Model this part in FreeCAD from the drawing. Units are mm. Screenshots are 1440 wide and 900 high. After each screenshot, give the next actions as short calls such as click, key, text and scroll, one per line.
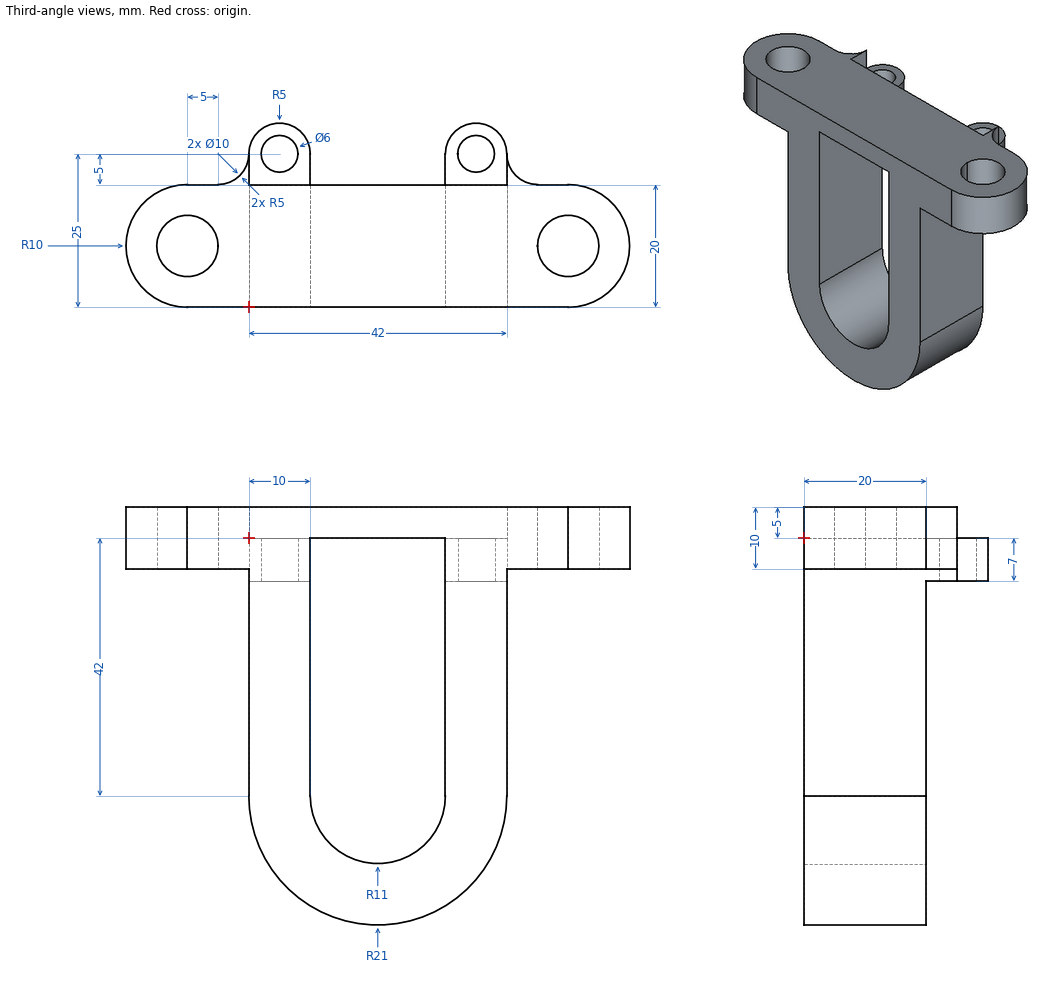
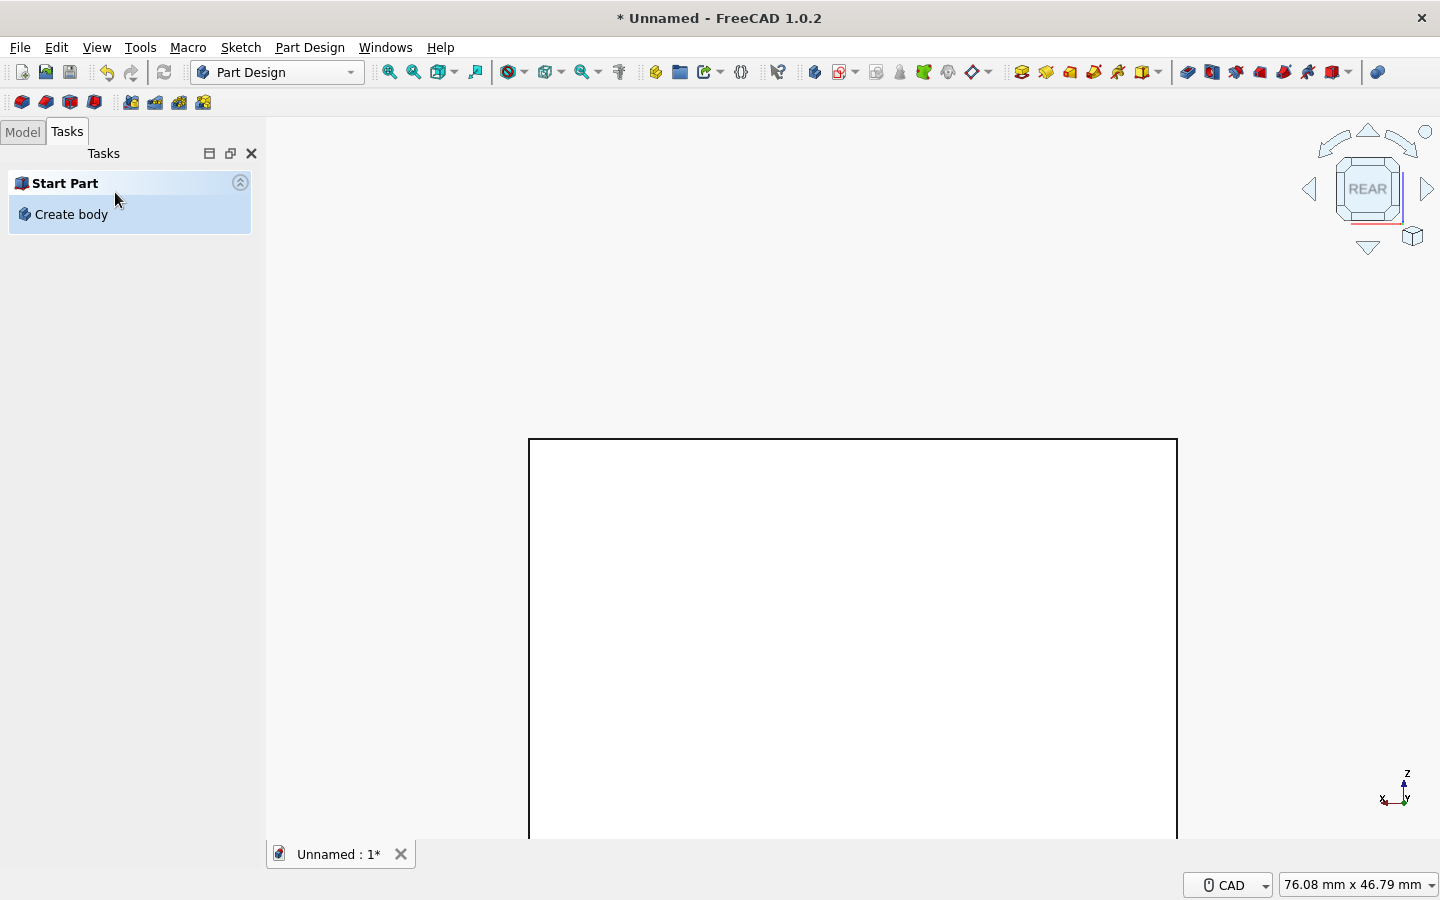
click(390, 72)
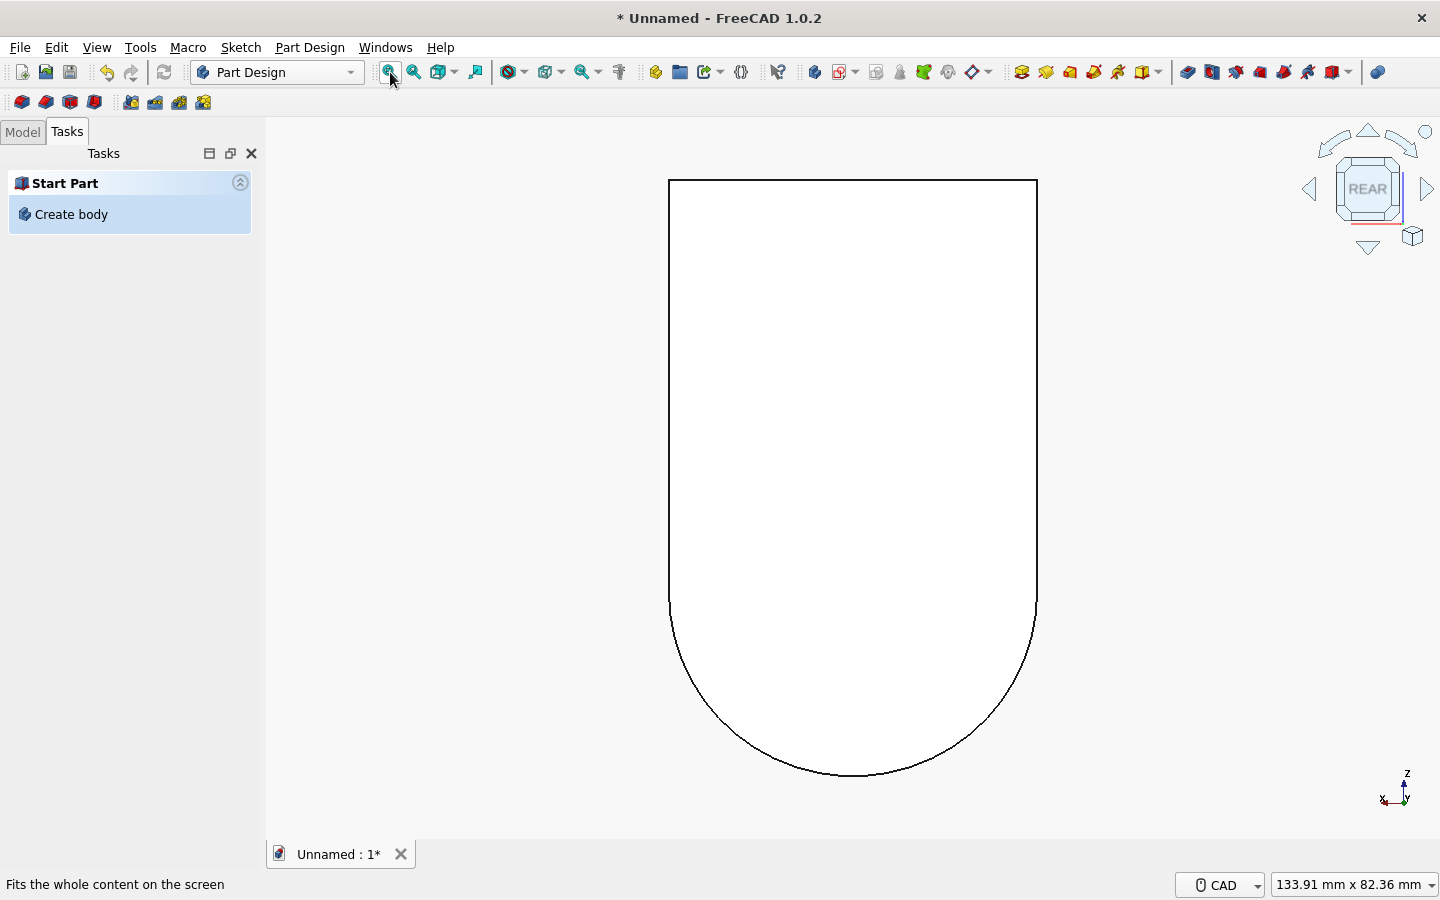
click(853, 392)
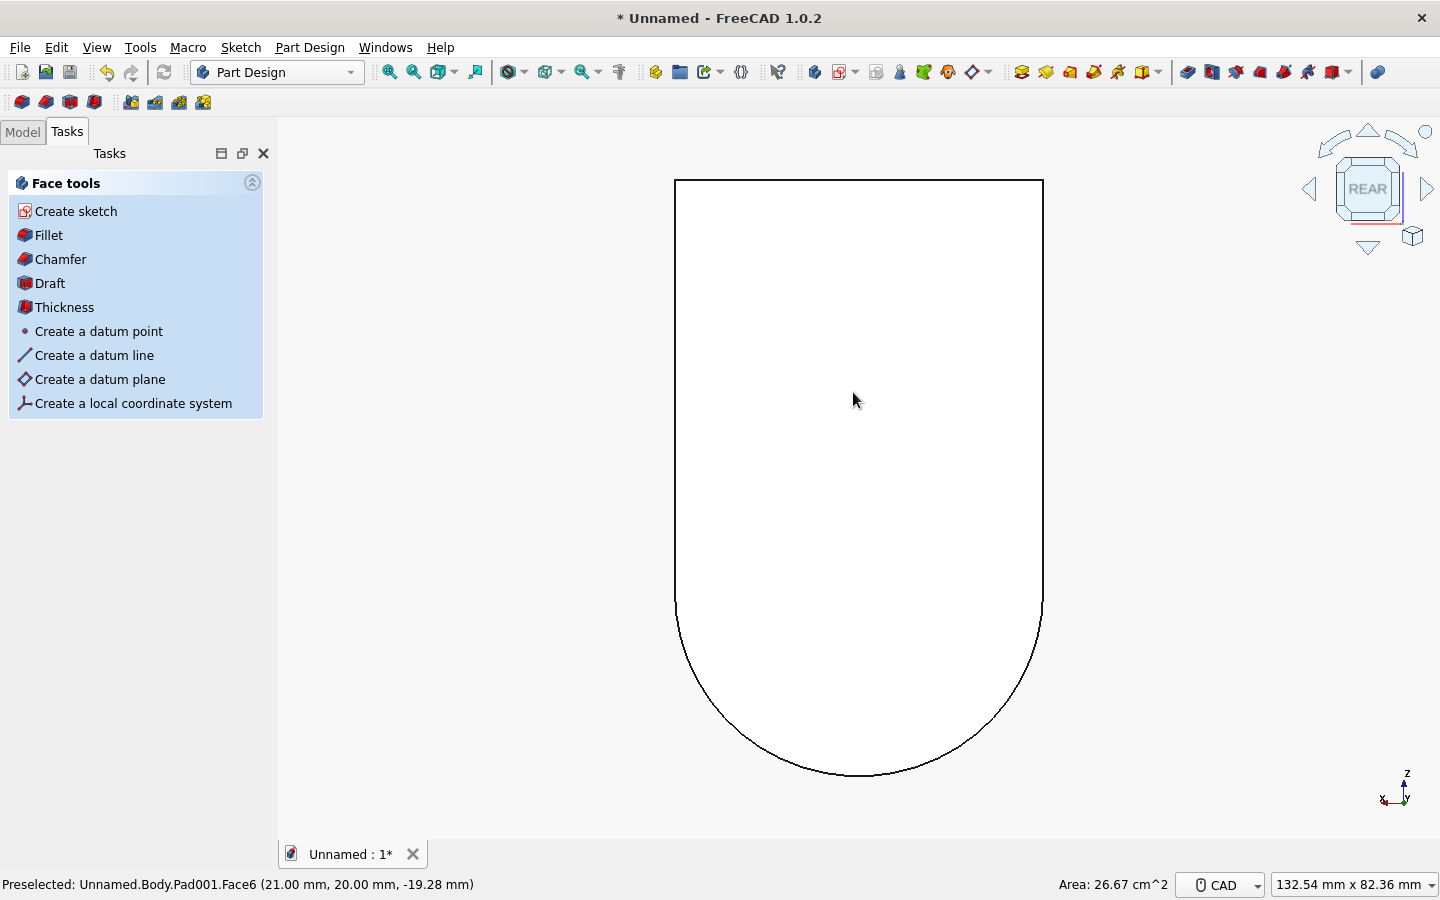
click(840, 72)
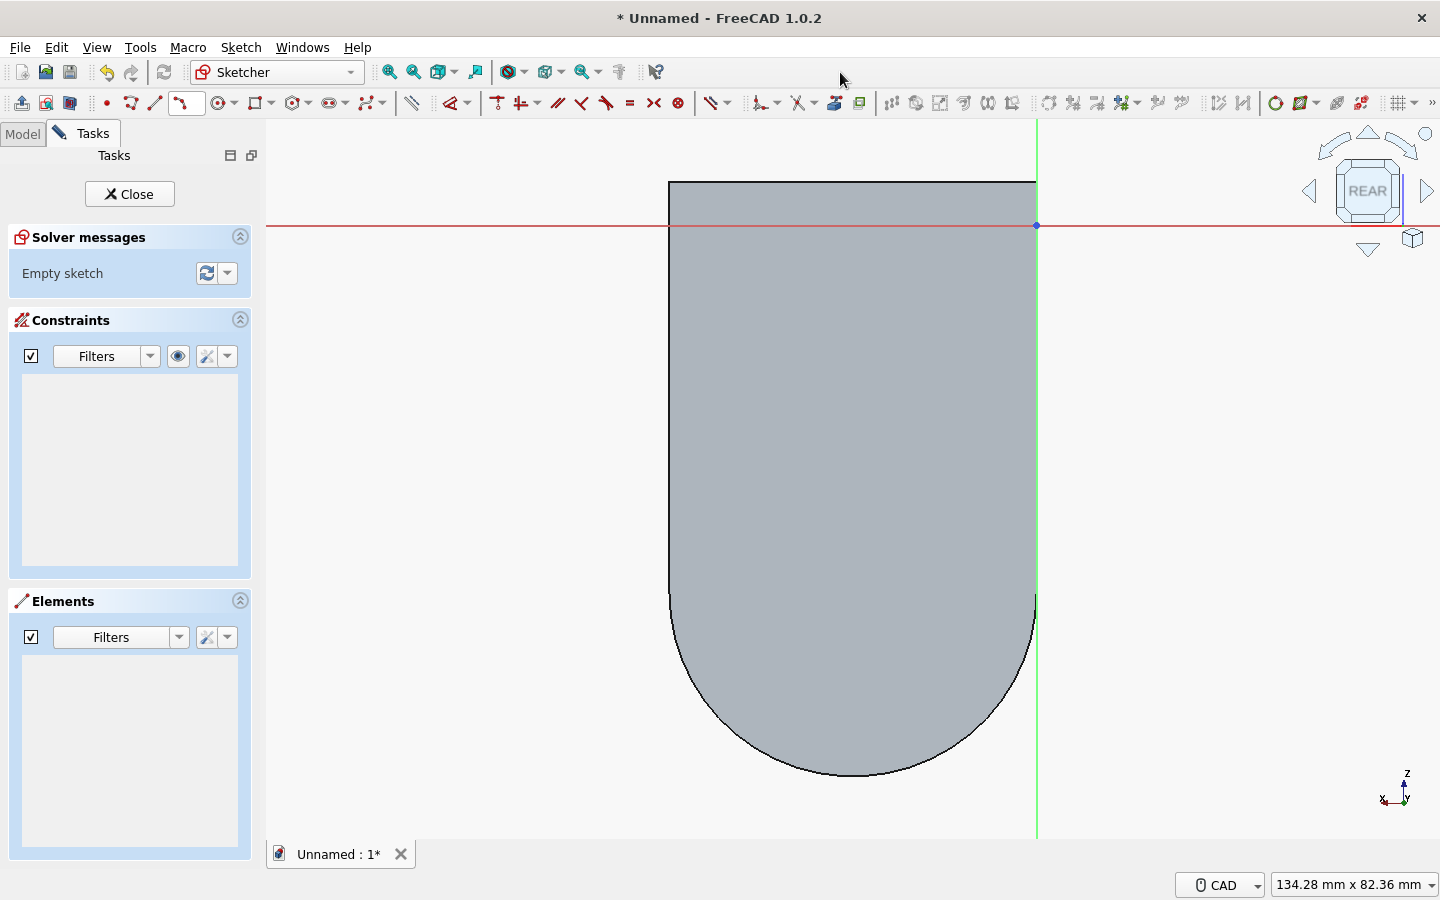
click(132, 104)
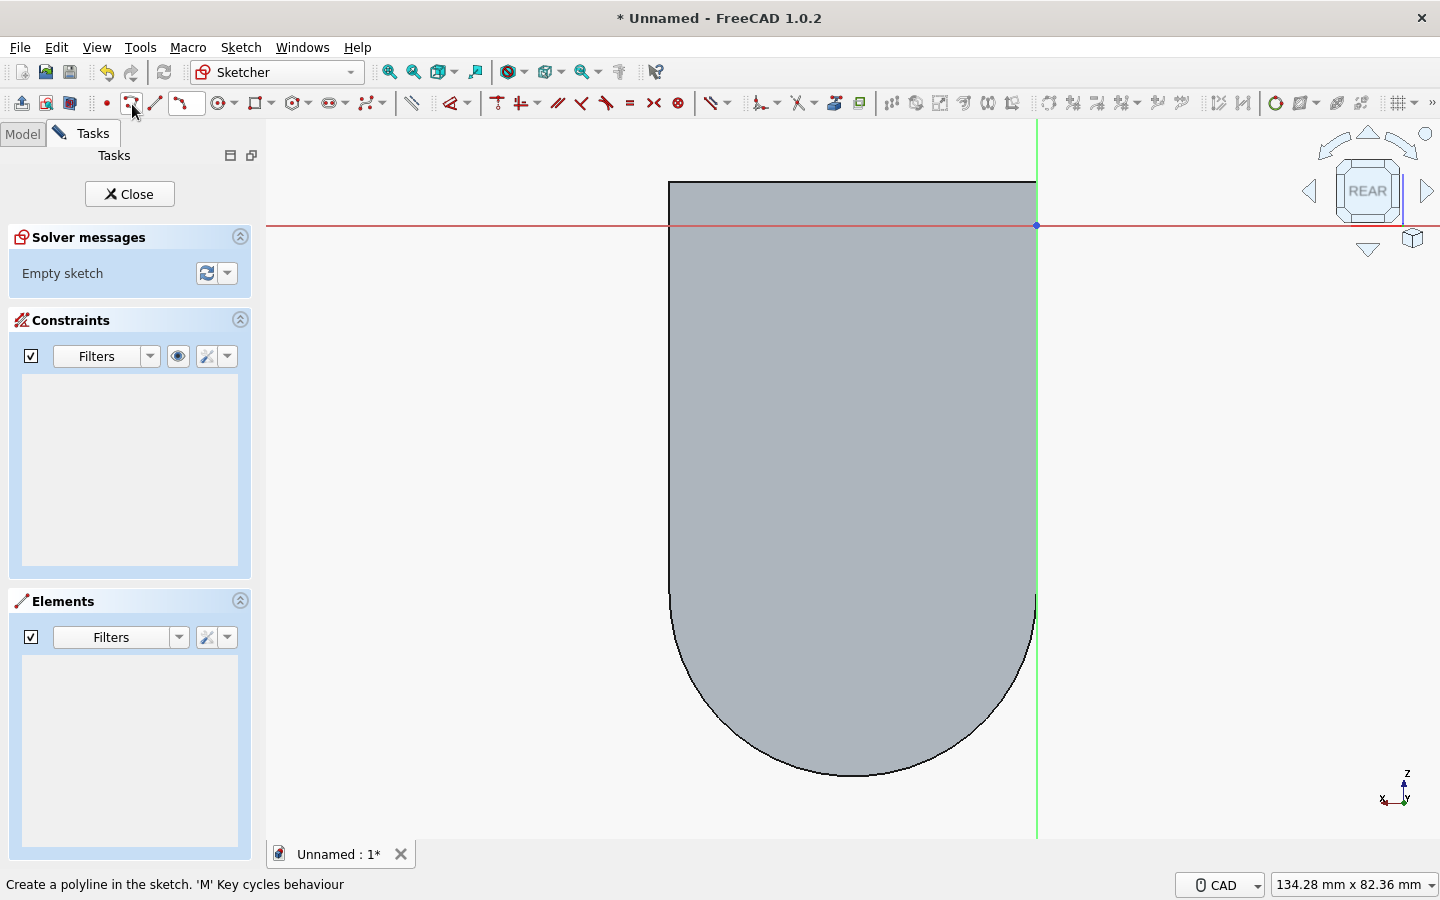
click(949, 593)
click(949, 226)
click(757, 235)
click(757, 593)
right_click(757, 593)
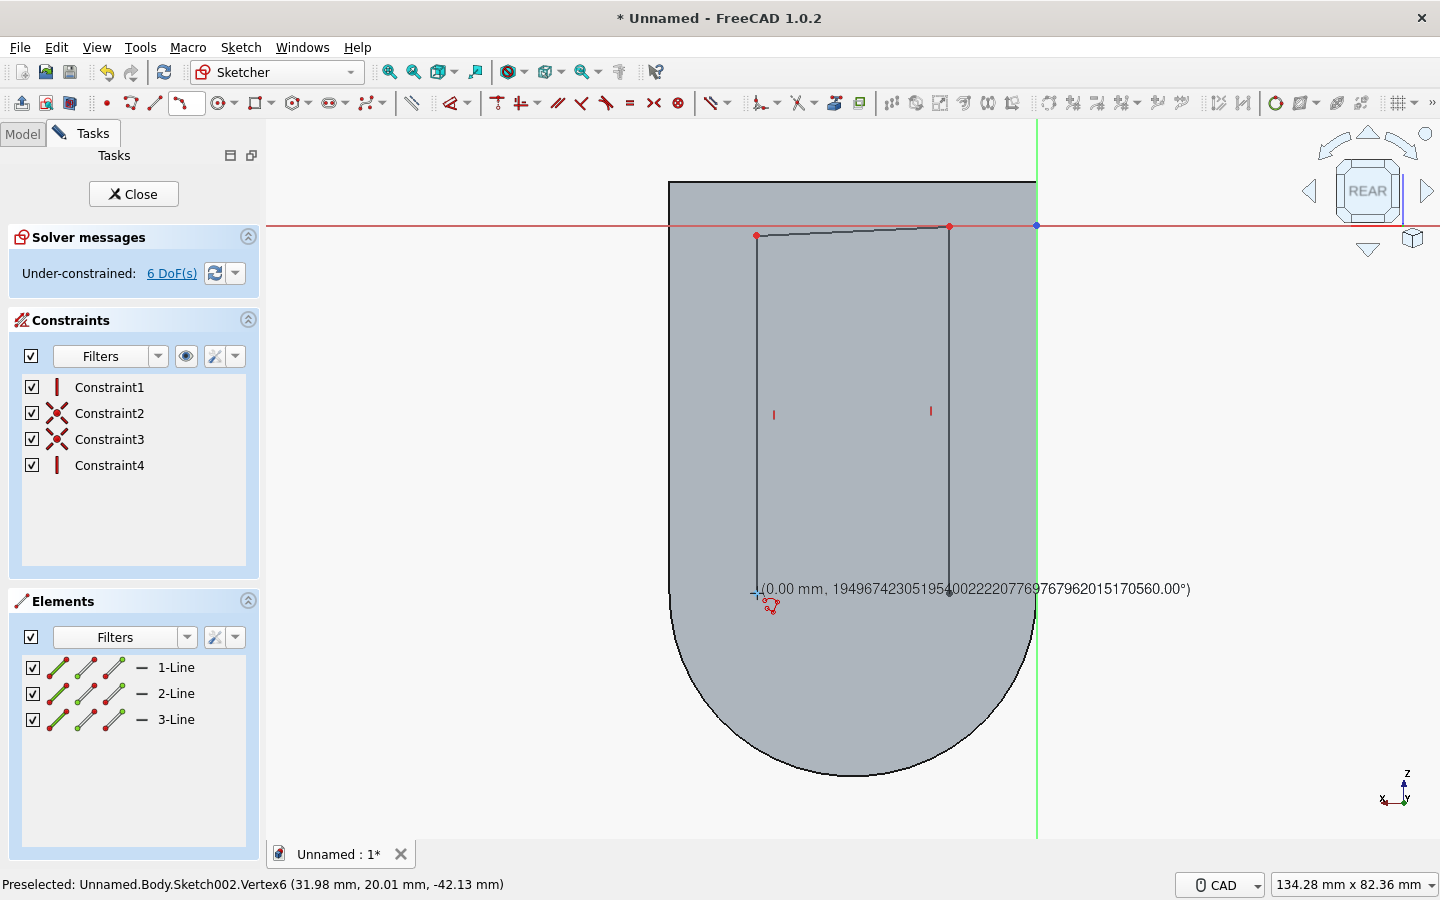
click(180, 104)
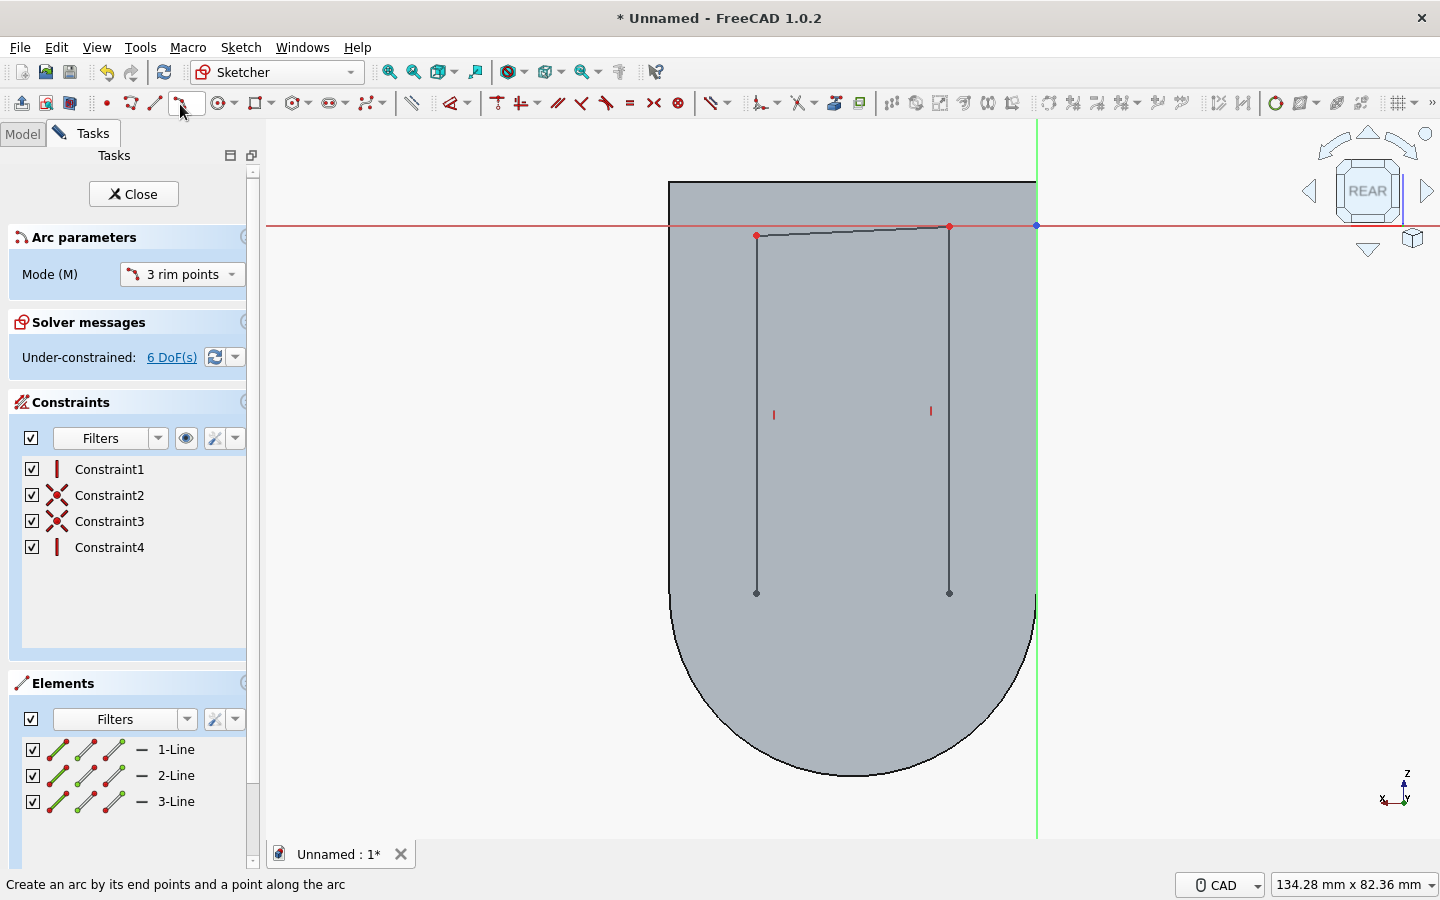
click(757, 594)
click(949, 594)
click(853, 689)
key(Escape)